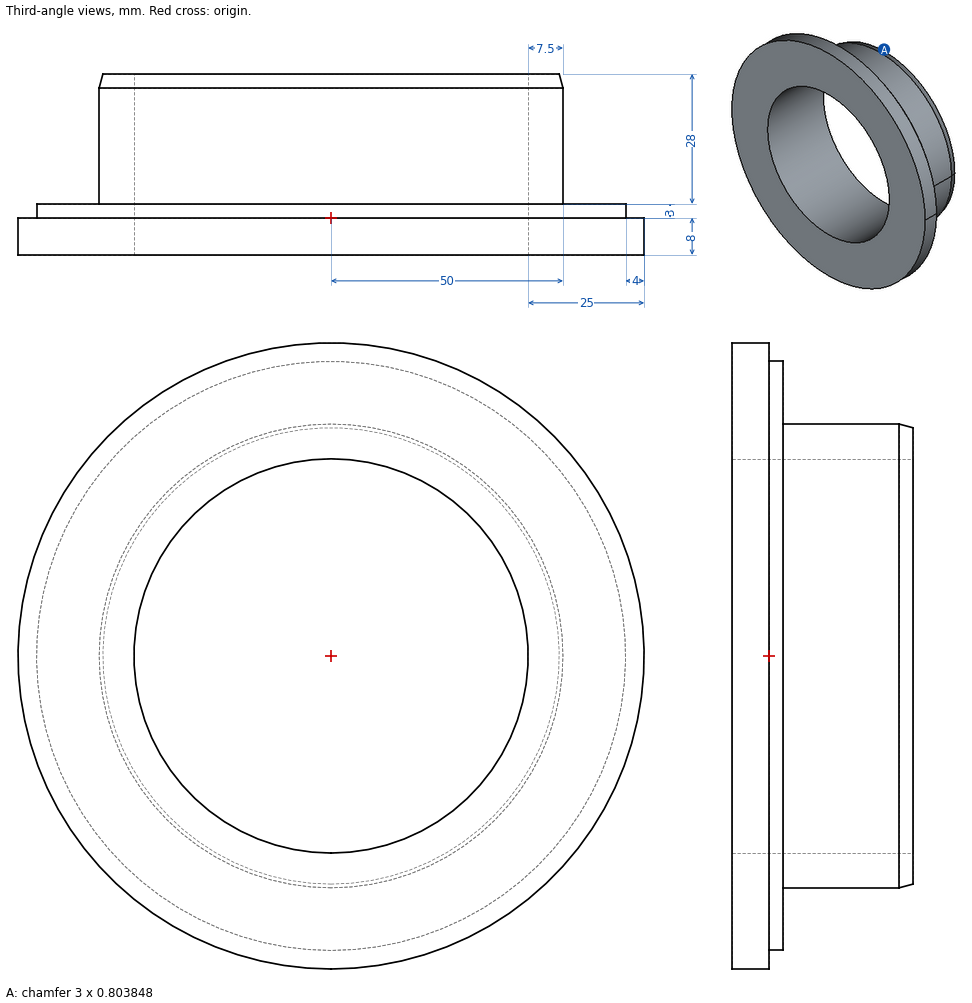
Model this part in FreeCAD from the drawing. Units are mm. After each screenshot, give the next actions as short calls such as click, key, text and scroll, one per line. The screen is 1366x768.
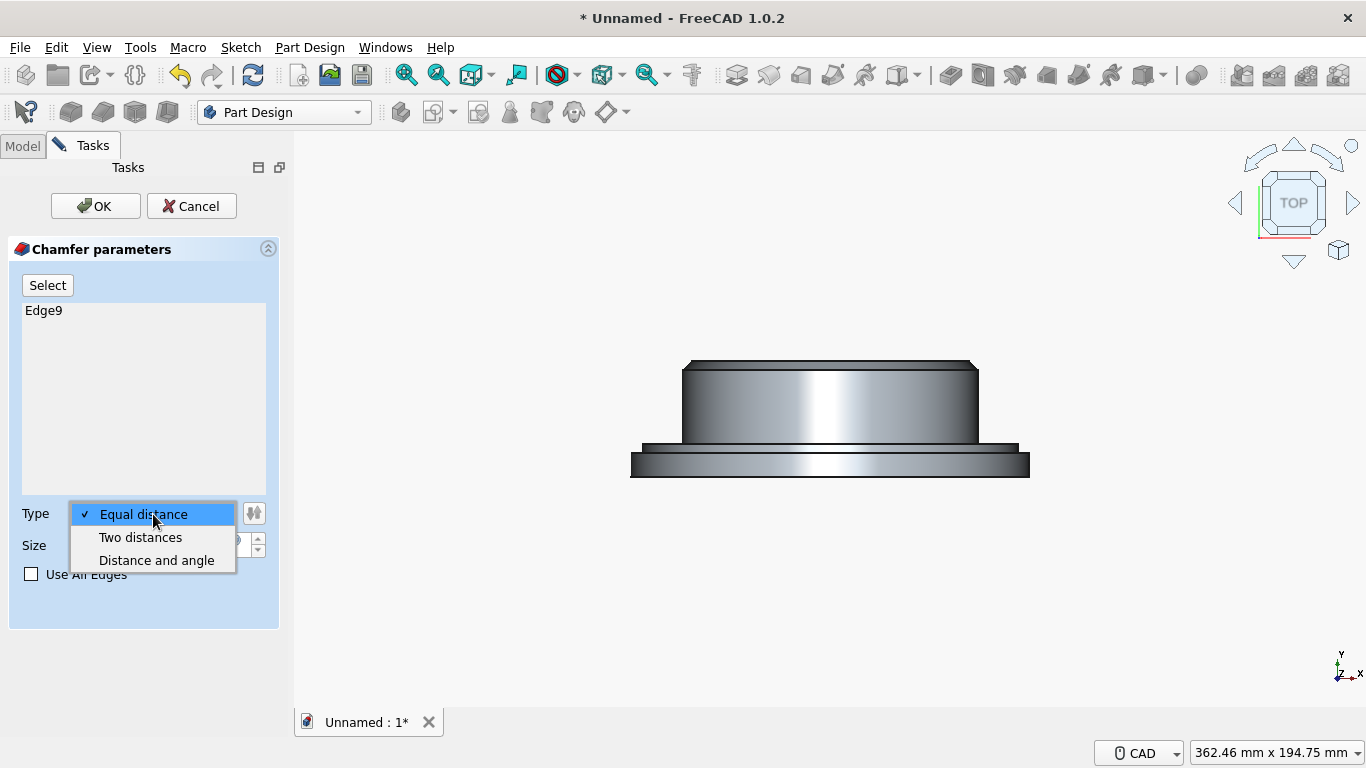
click(152, 538)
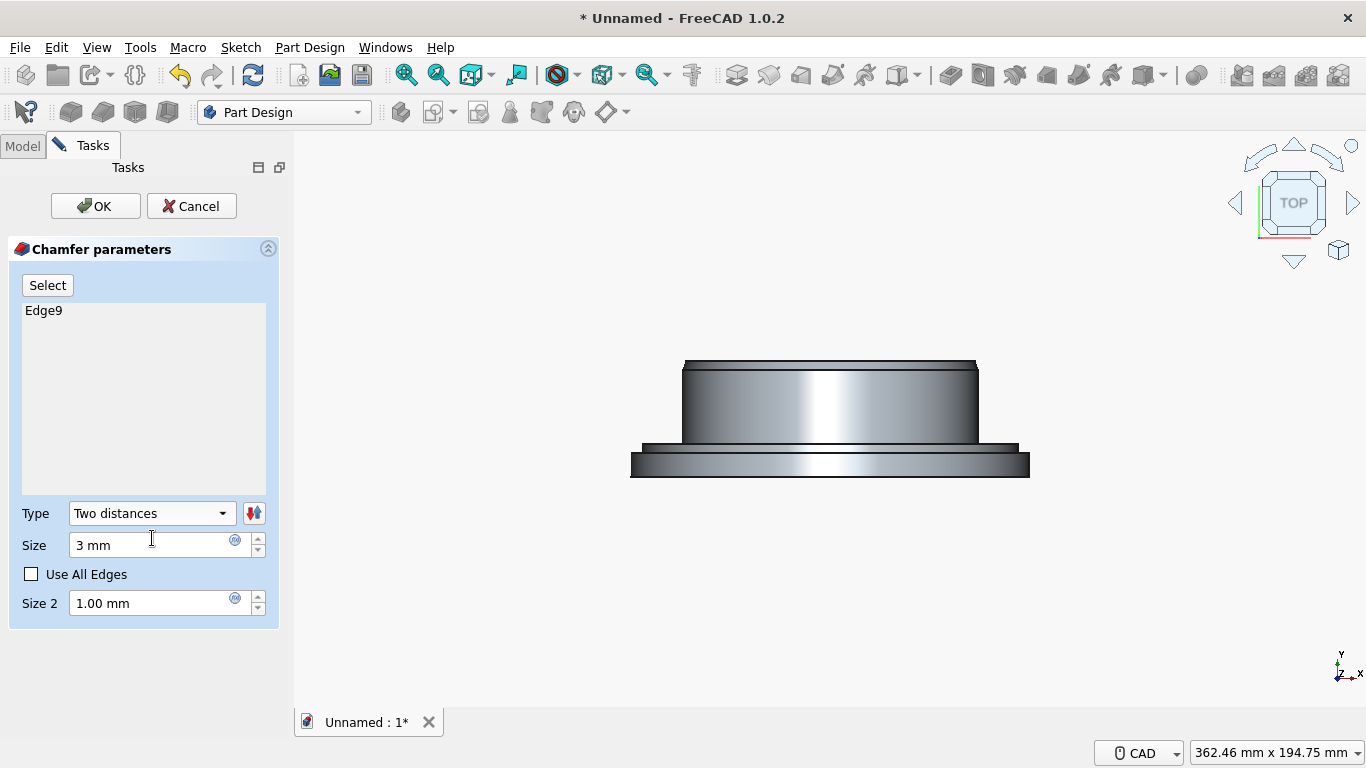
triple_click(160, 603)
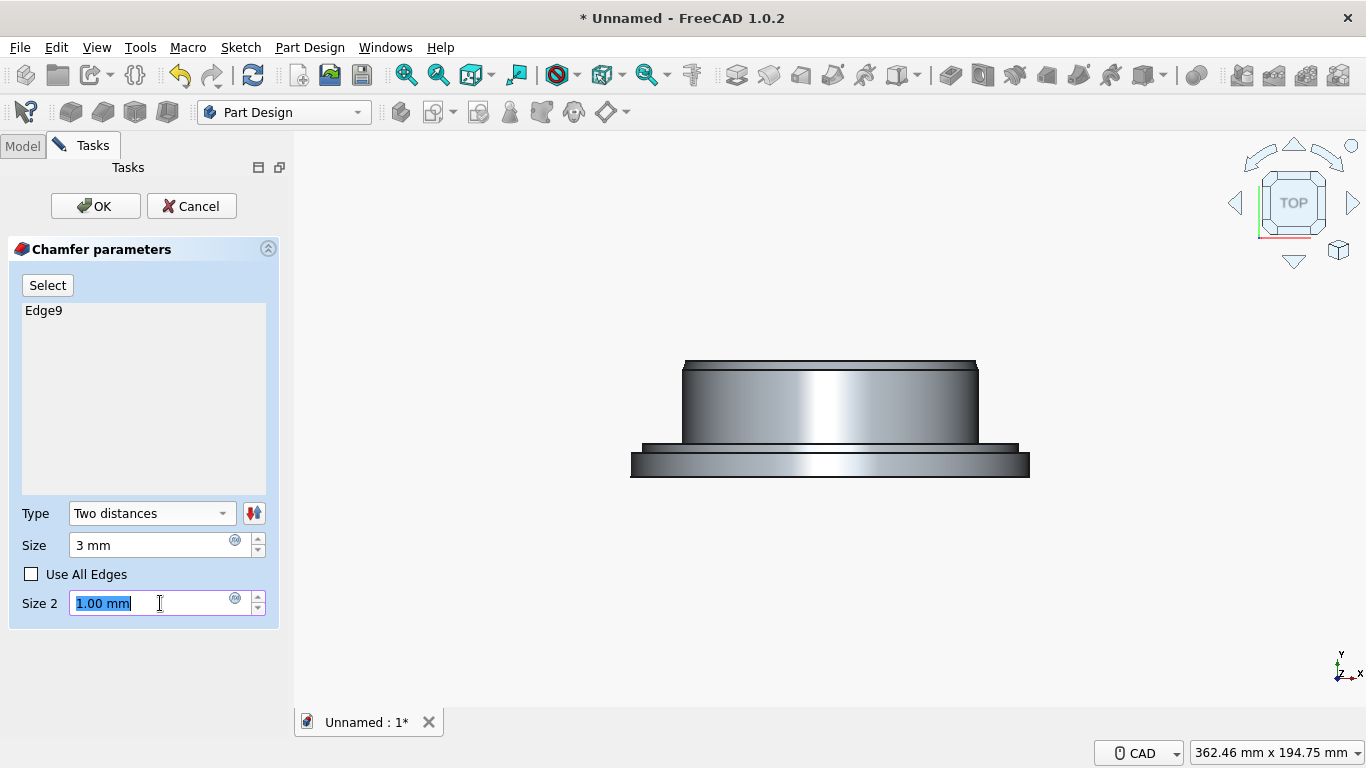
text(0.803848)
key(Tab)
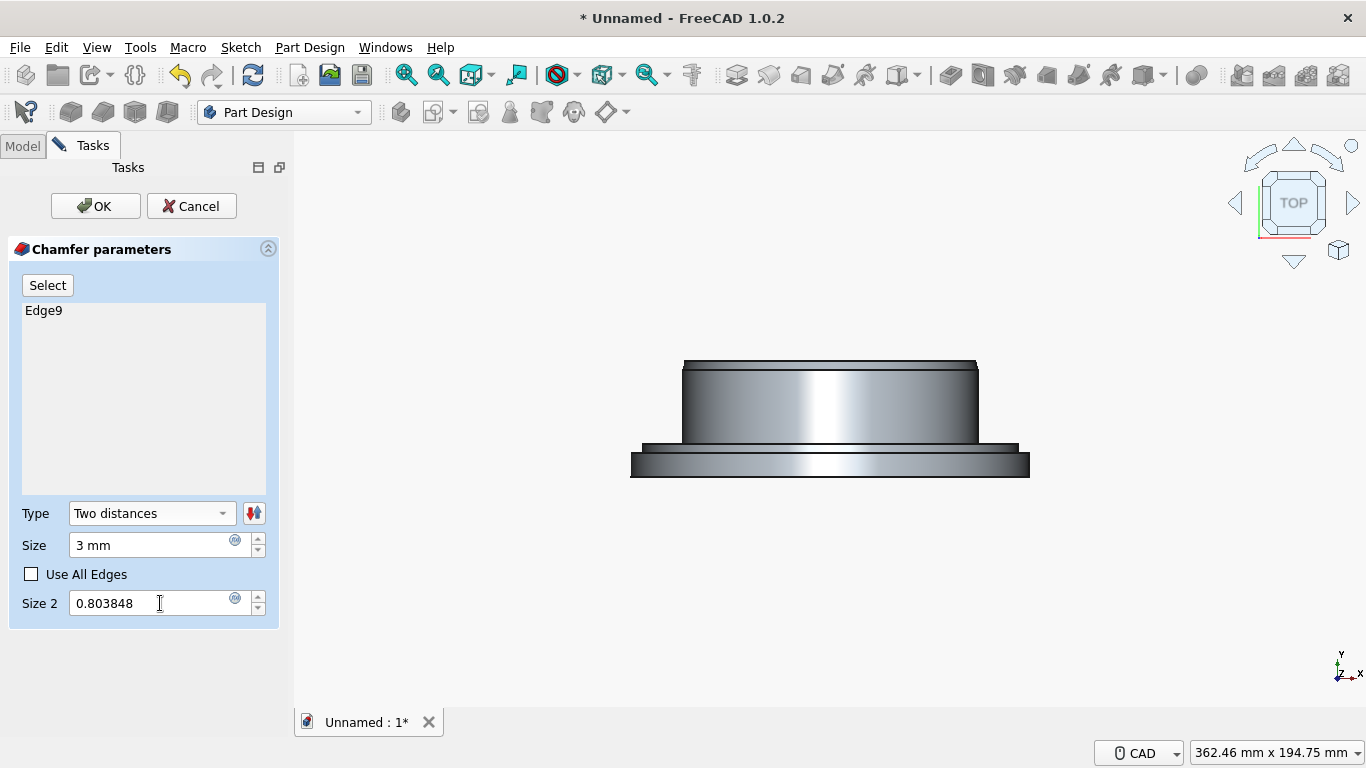
click(96, 206)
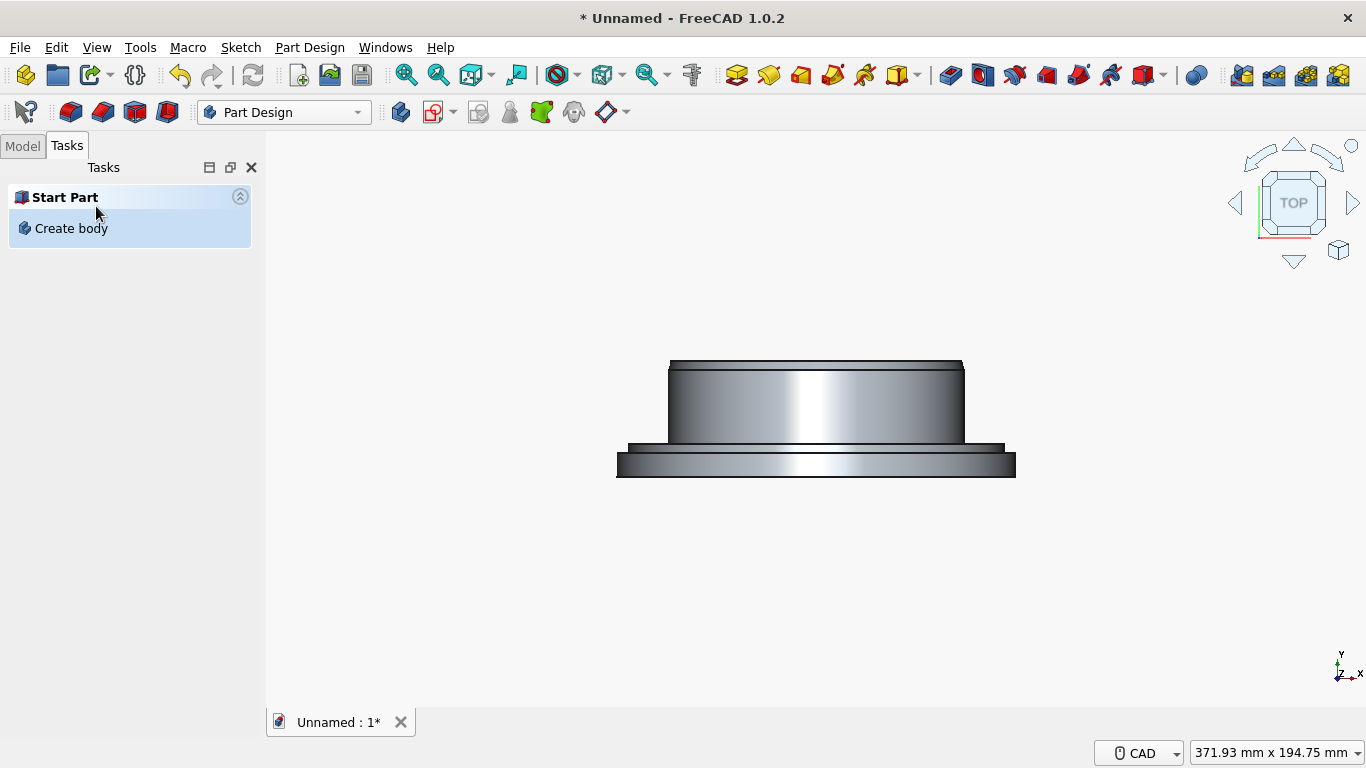
key(0)